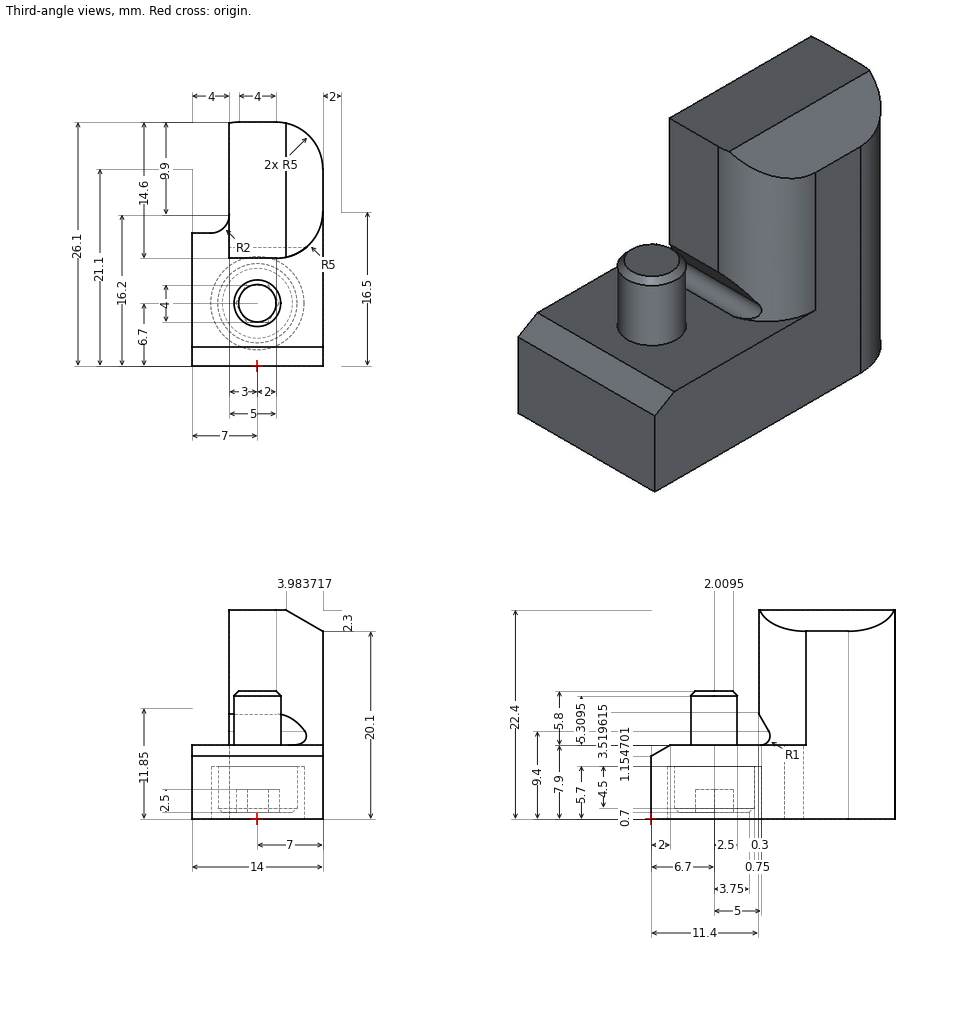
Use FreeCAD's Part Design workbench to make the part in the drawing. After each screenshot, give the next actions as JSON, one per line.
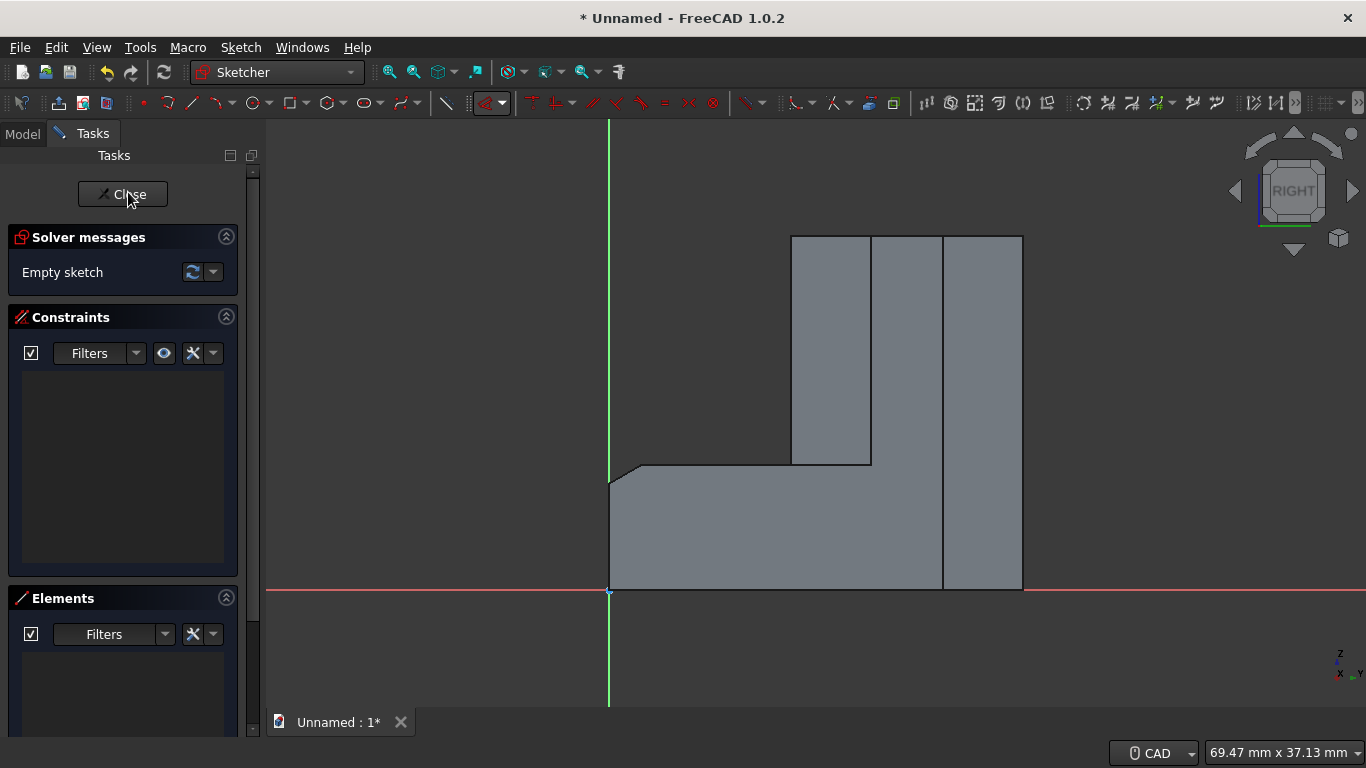
{"action": "left_click", "coordinate": [108, 104]}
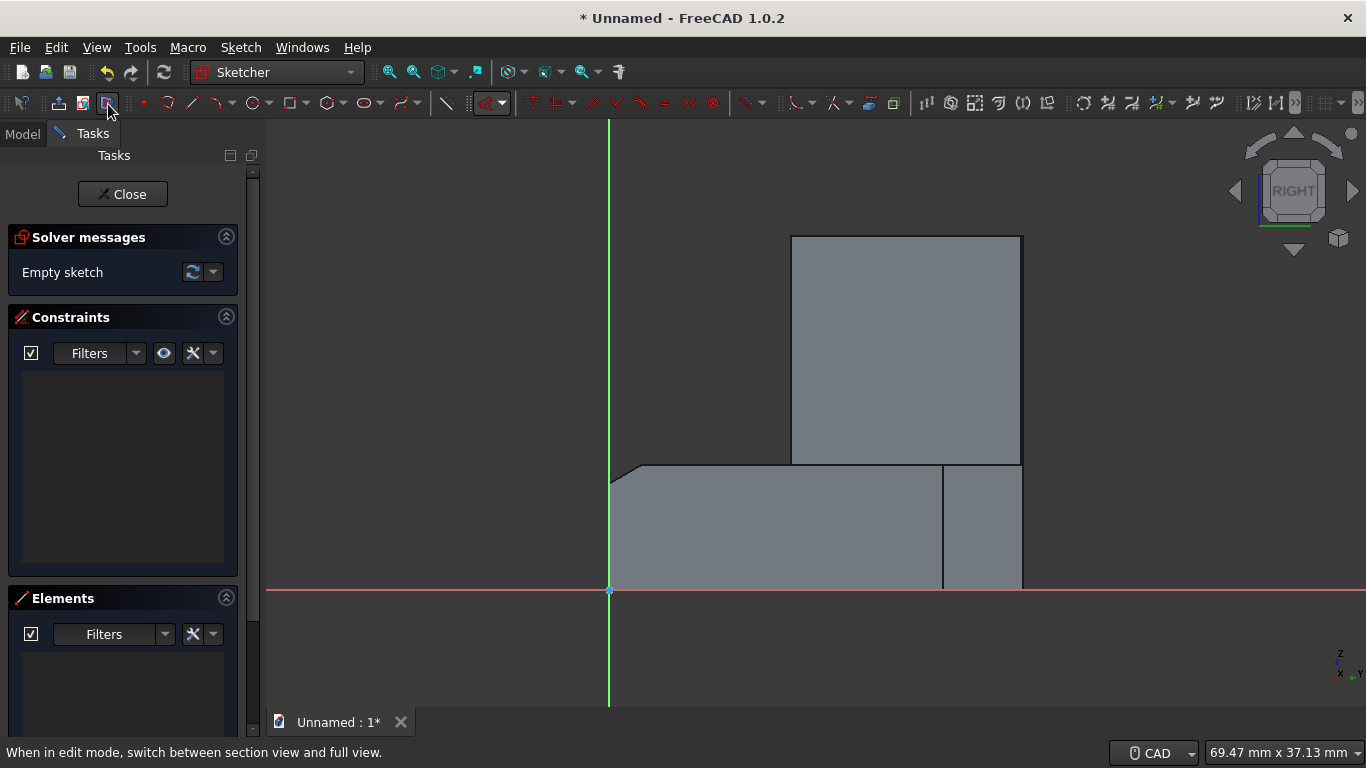
{"action": "scroll", "coordinate": [676, 594], "scroll_direction": "up", "scroll_amount": 5}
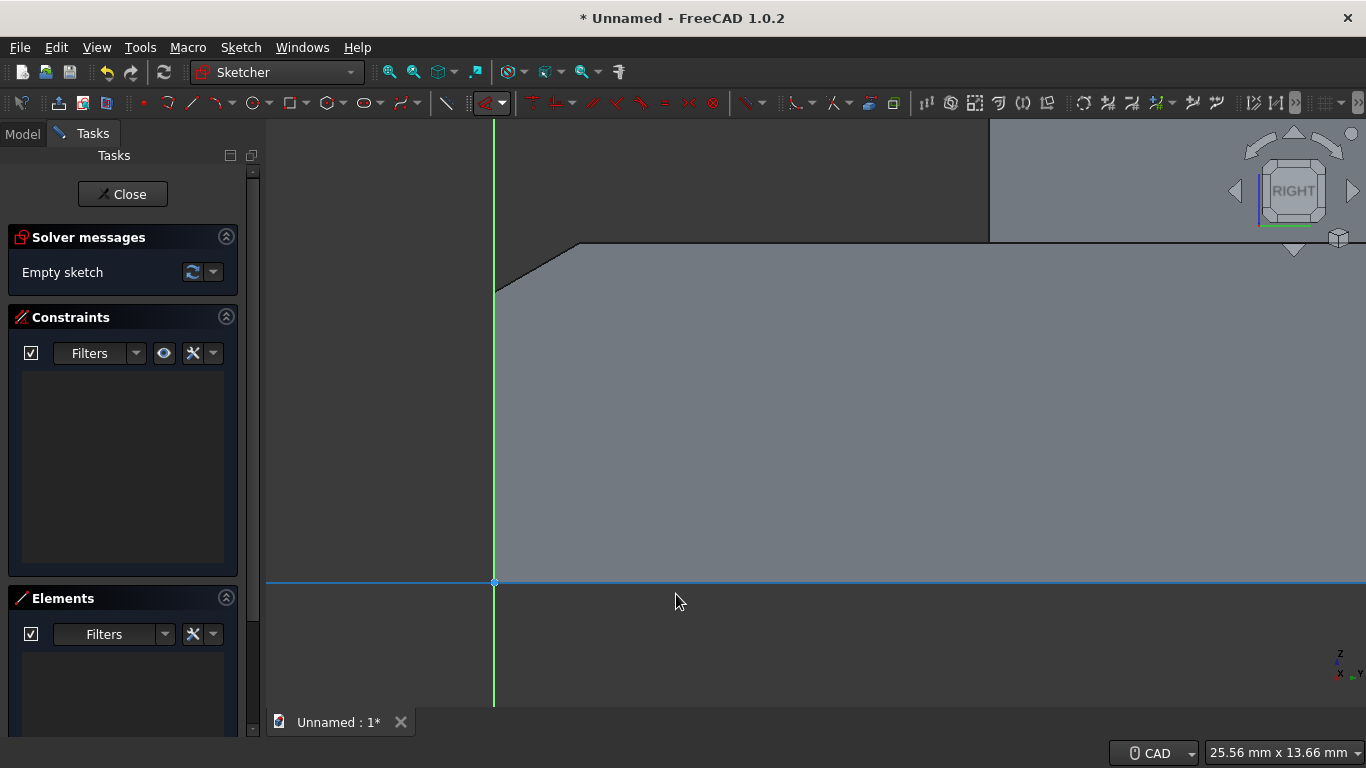
{"action": "left_click", "coordinate": [168, 104]}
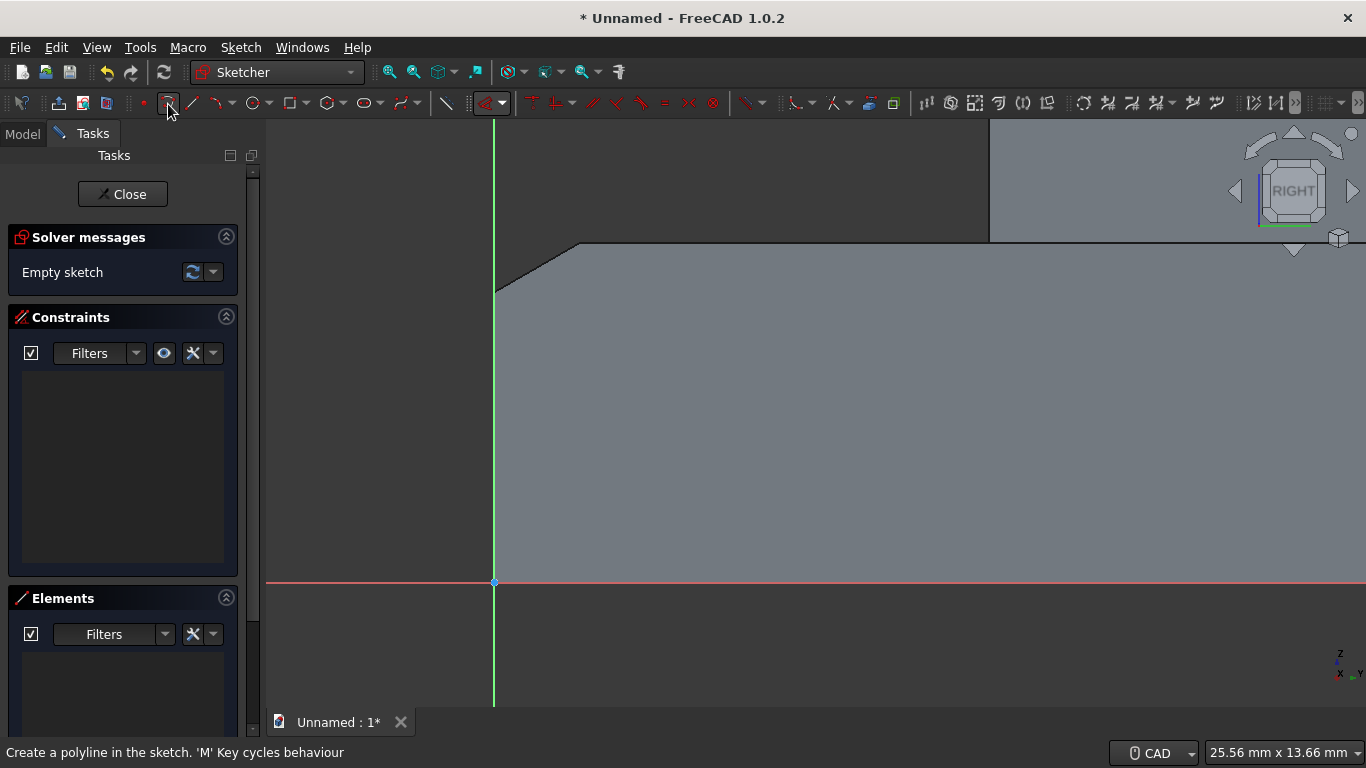
{"action": "left_click", "coordinate": [783, 583]}
{"action": "left_click", "coordinate": [998, 574]}
{"action": "left_click", "coordinate": [998, 337]}
{"action": "left_click", "coordinate": [966, 337]}
{"action": "left_click", "coordinate": [966, 531]}
{"action": "left_click", "coordinate": [944, 553]}
{"action": "left_click", "coordinate": [783, 553]}
{"action": "left_click", "coordinate": [783, 583]}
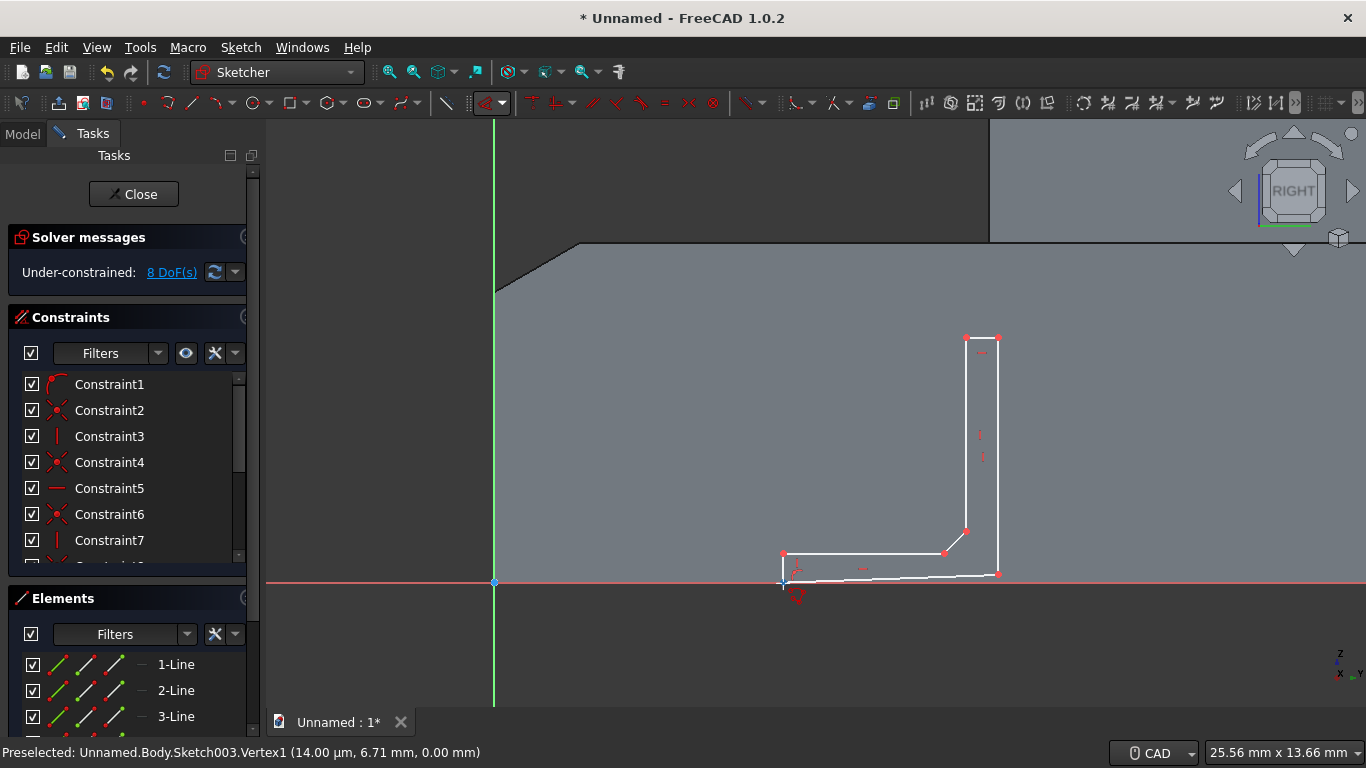
{"action": "left_click", "coordinate": [192, 104]}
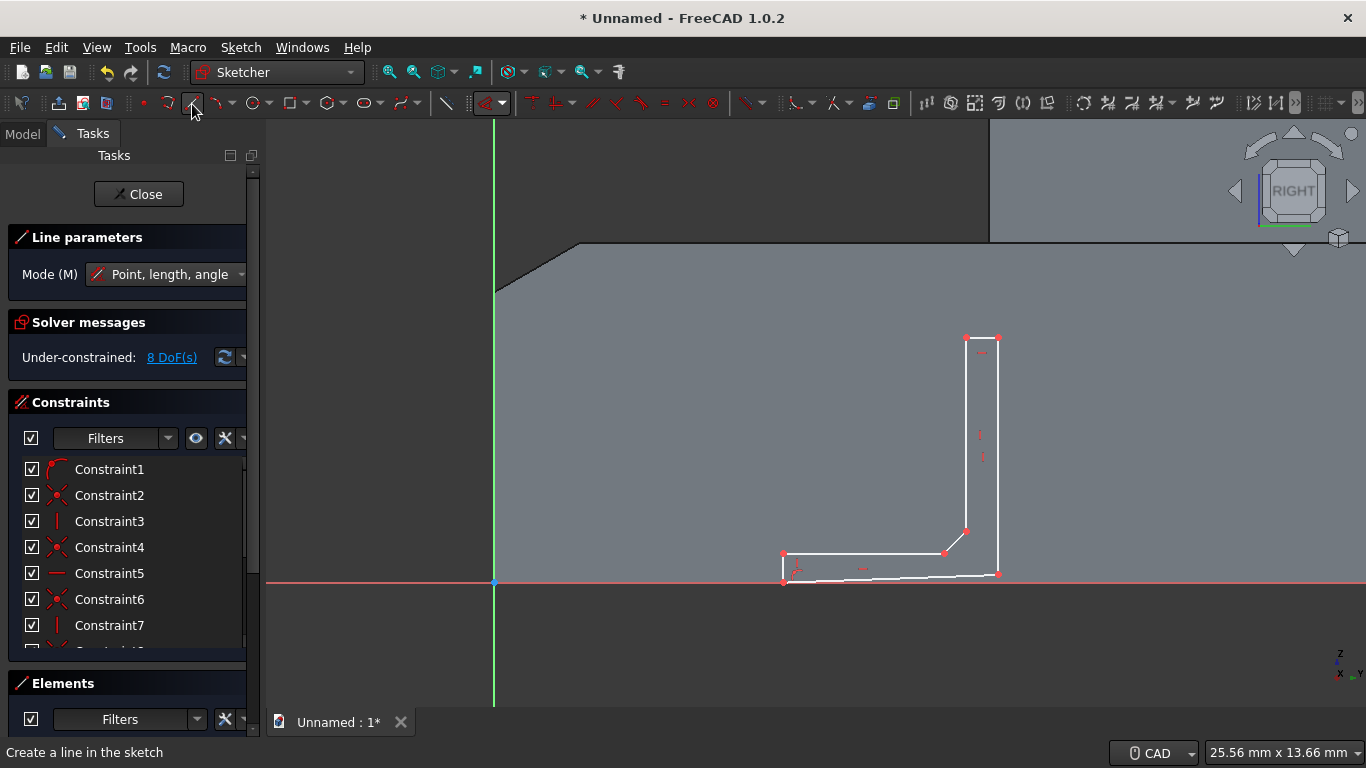
{"action": "left_click", "coordinate": [783, 313]}
{"action": "left_click", "coordinate": [783, 239]}
{"action": "key", "text": "Escape"}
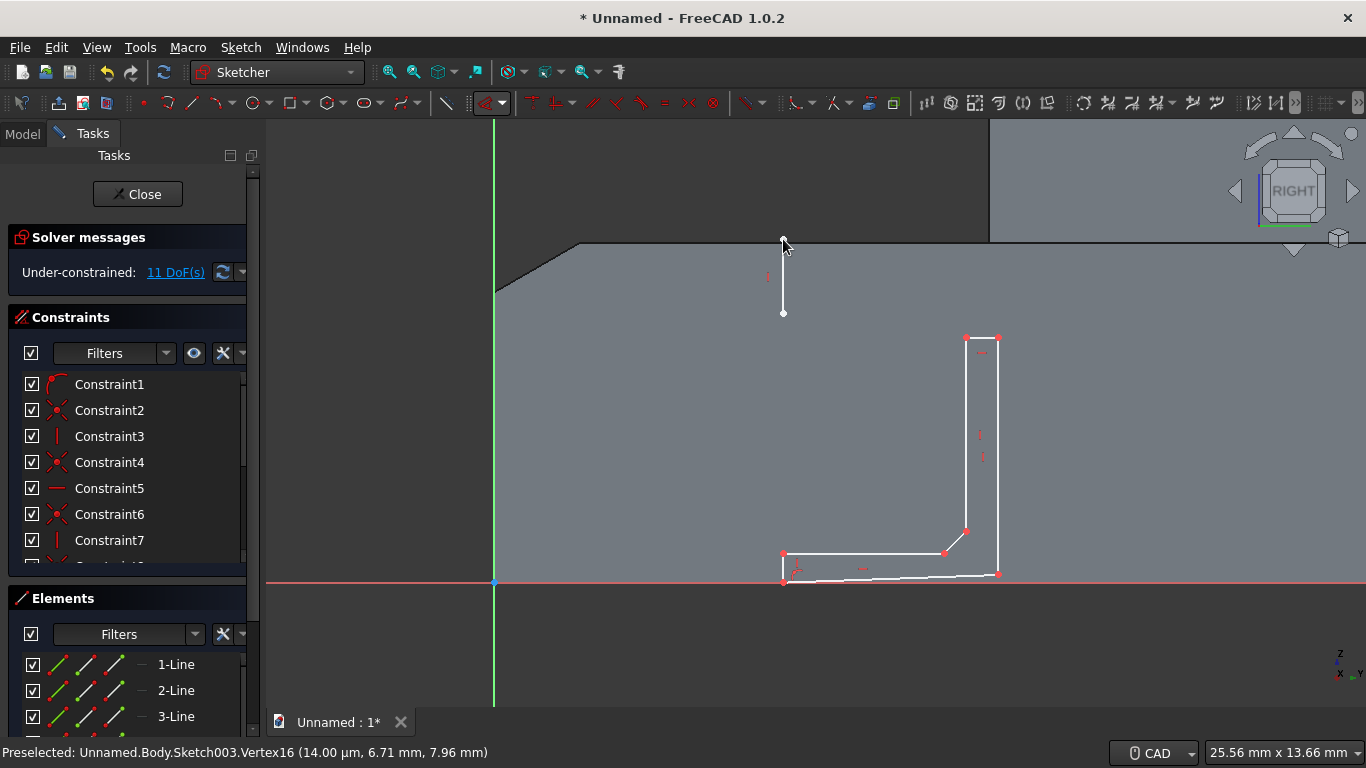
{"action": "left_click", "coordinate": [783, 292]}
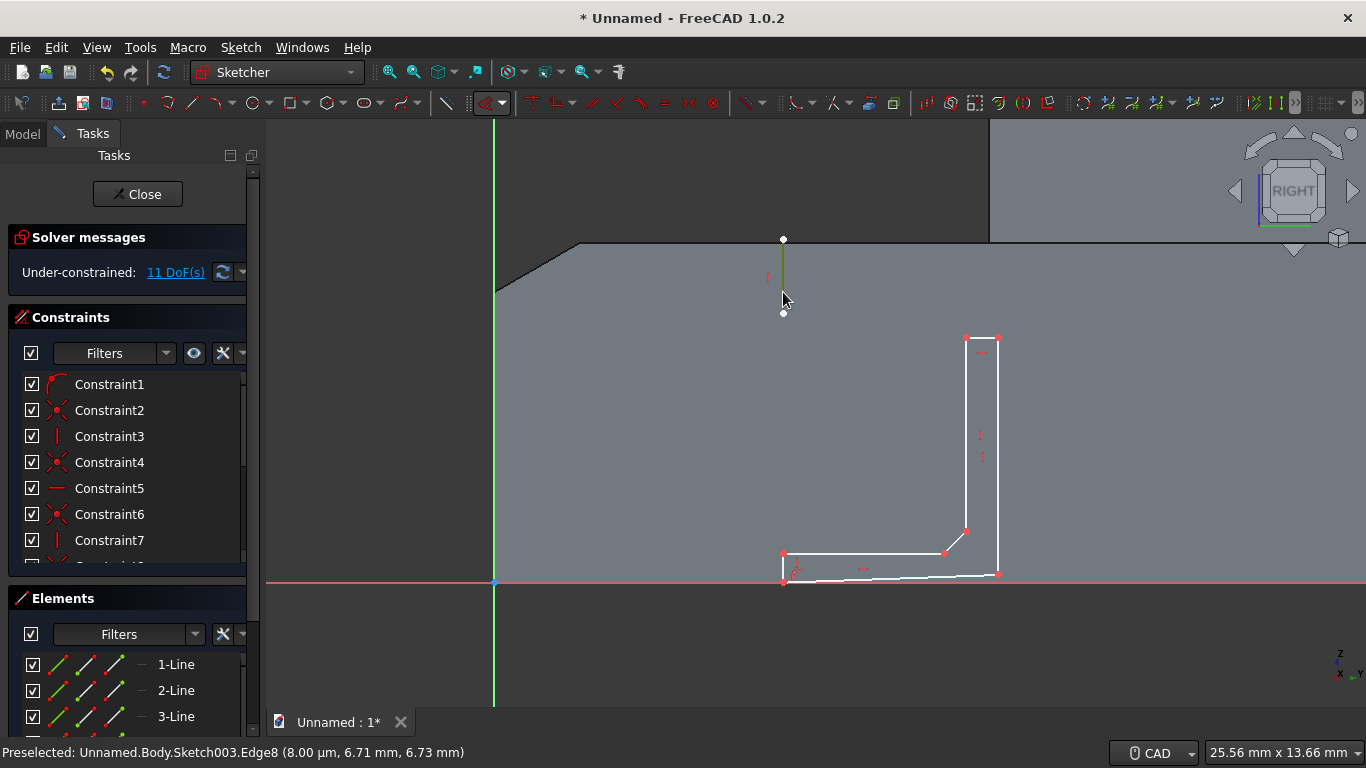
{"action": "left_click", "coordinate": [448, 104]}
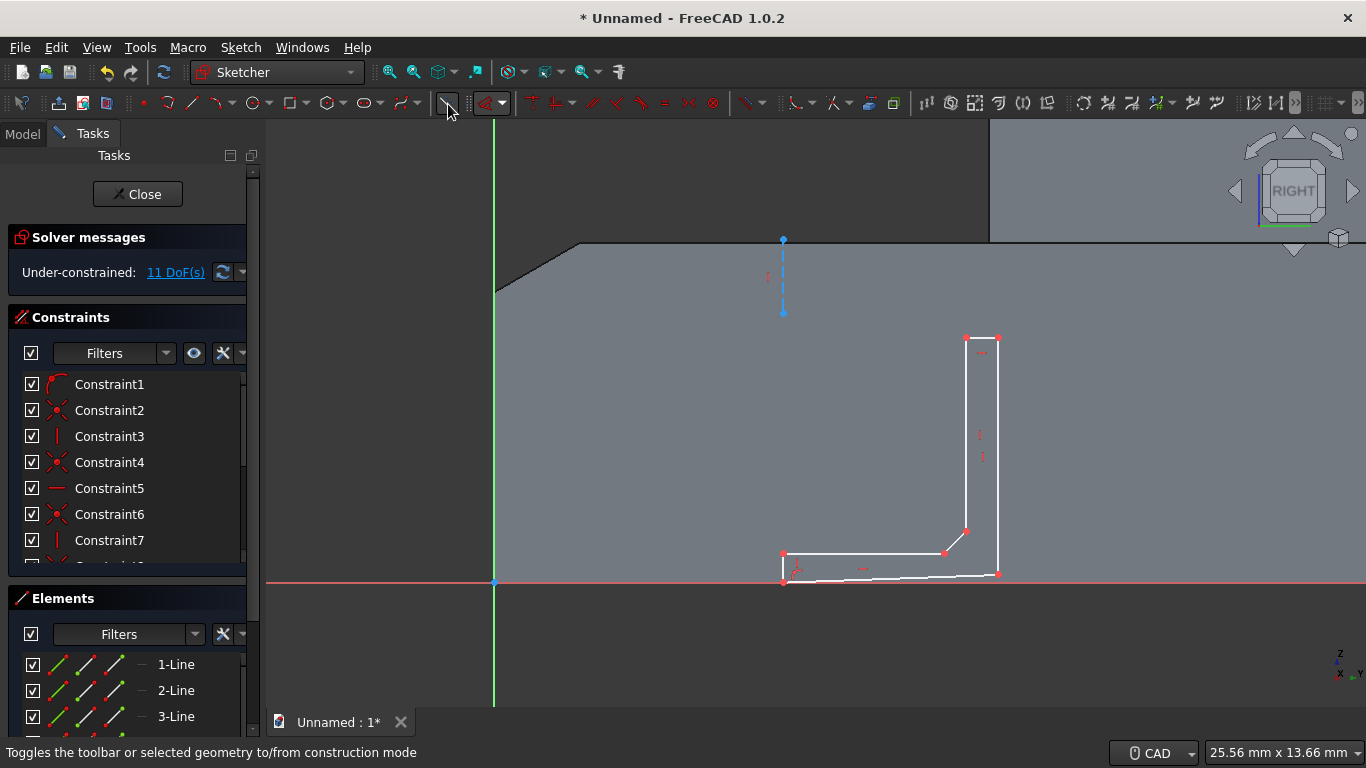
{"action": "left_click", "coordinate": [847, 580]}